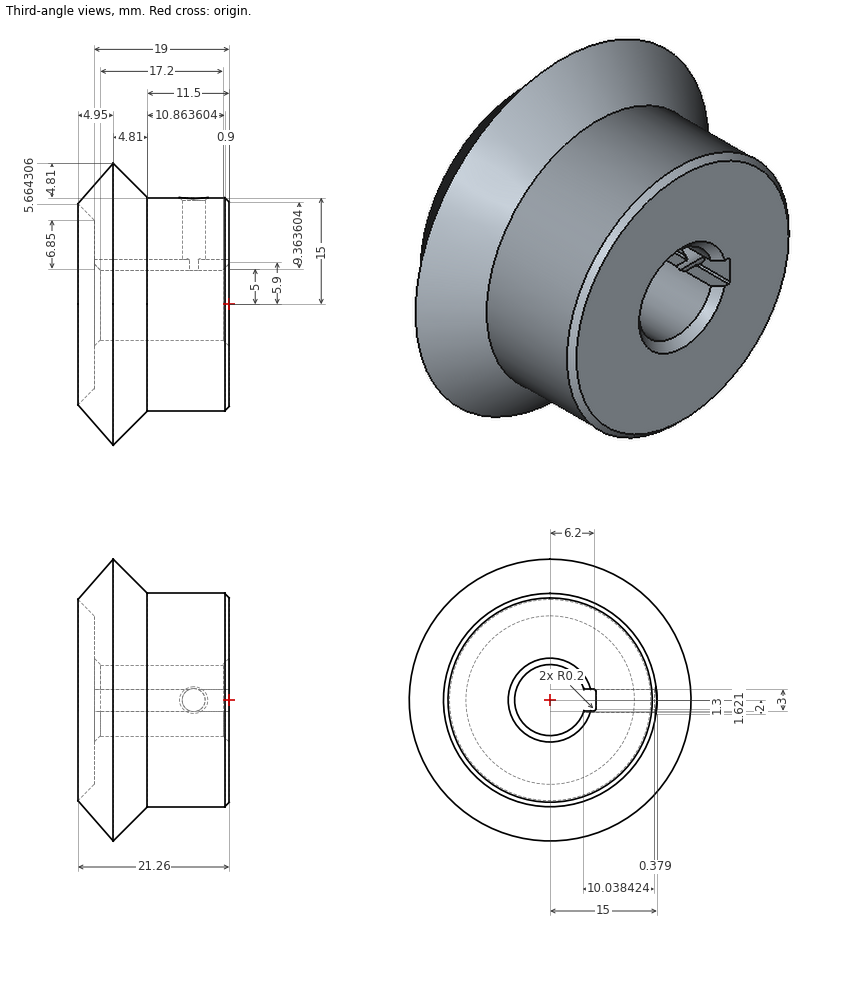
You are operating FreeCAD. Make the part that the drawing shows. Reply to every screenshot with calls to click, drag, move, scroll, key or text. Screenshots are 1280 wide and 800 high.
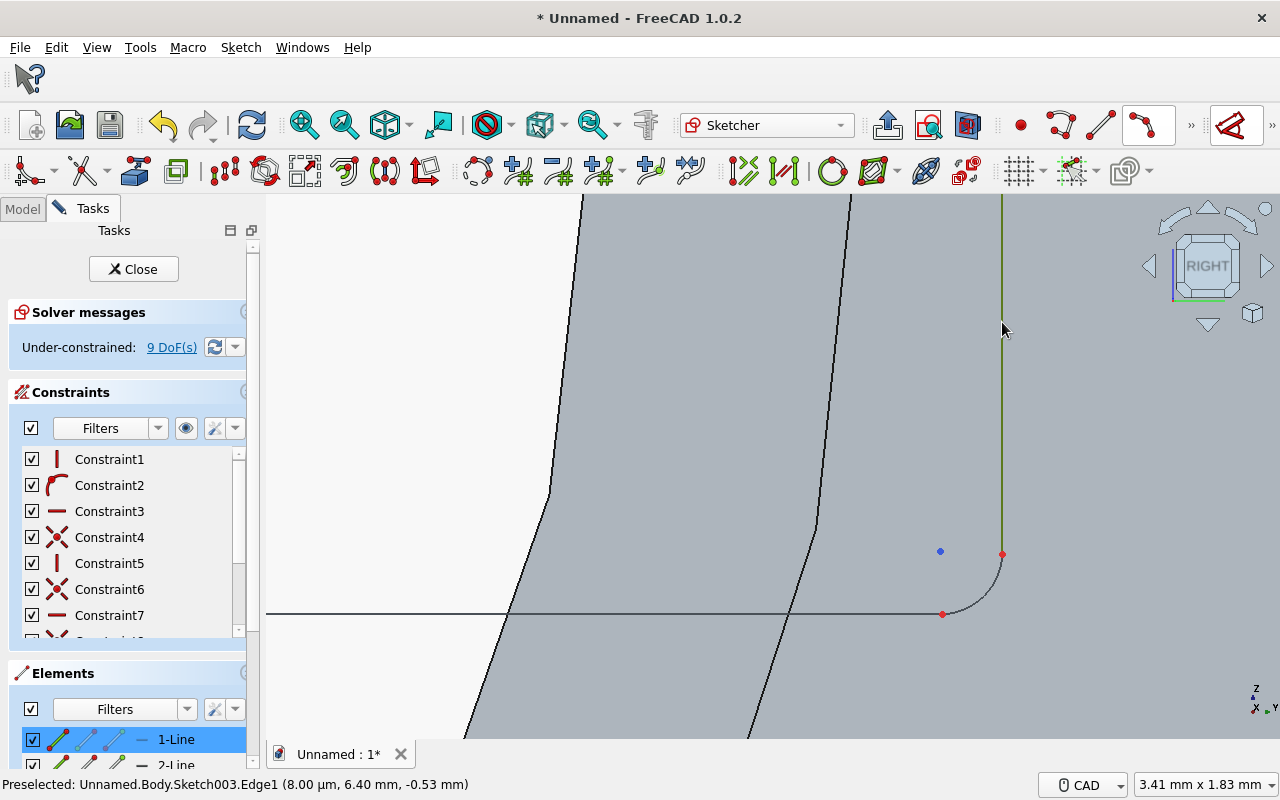
scroll(986, 597, down, 6)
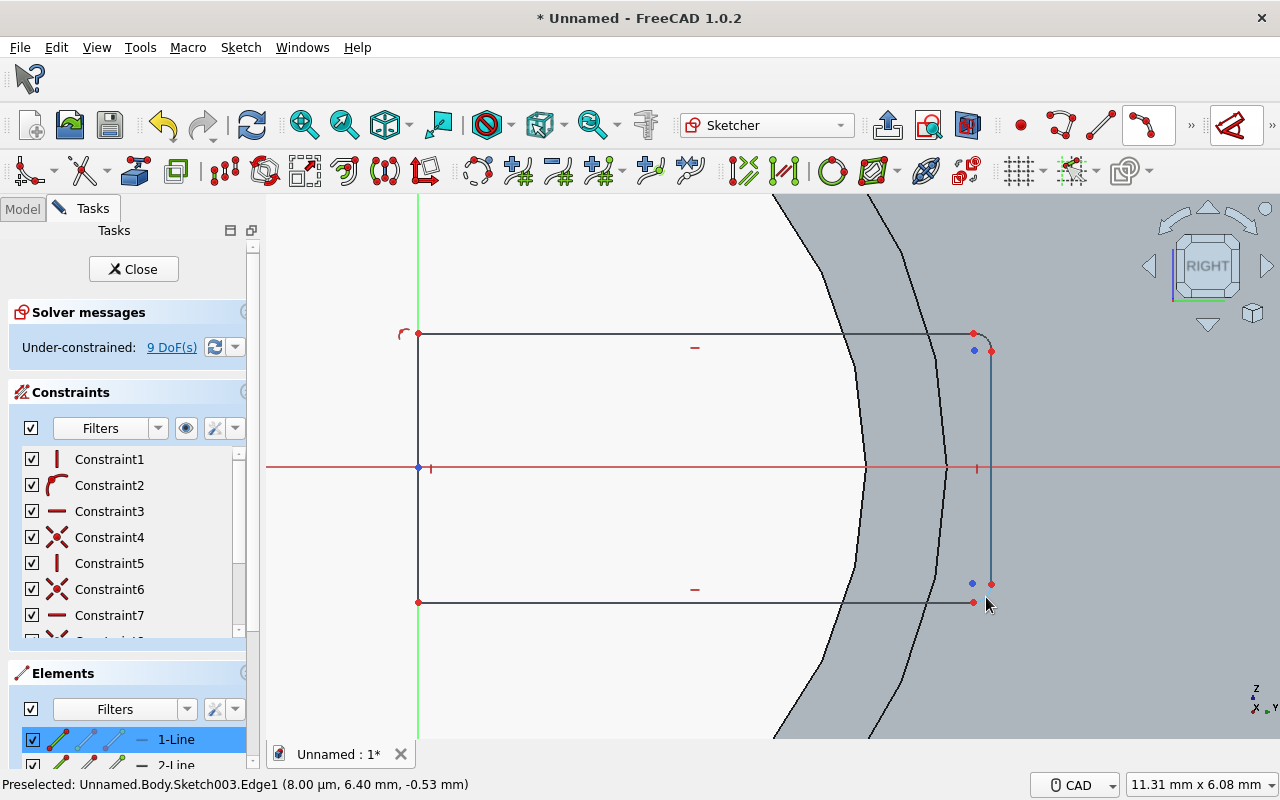
scroll(990, 343, up, 3)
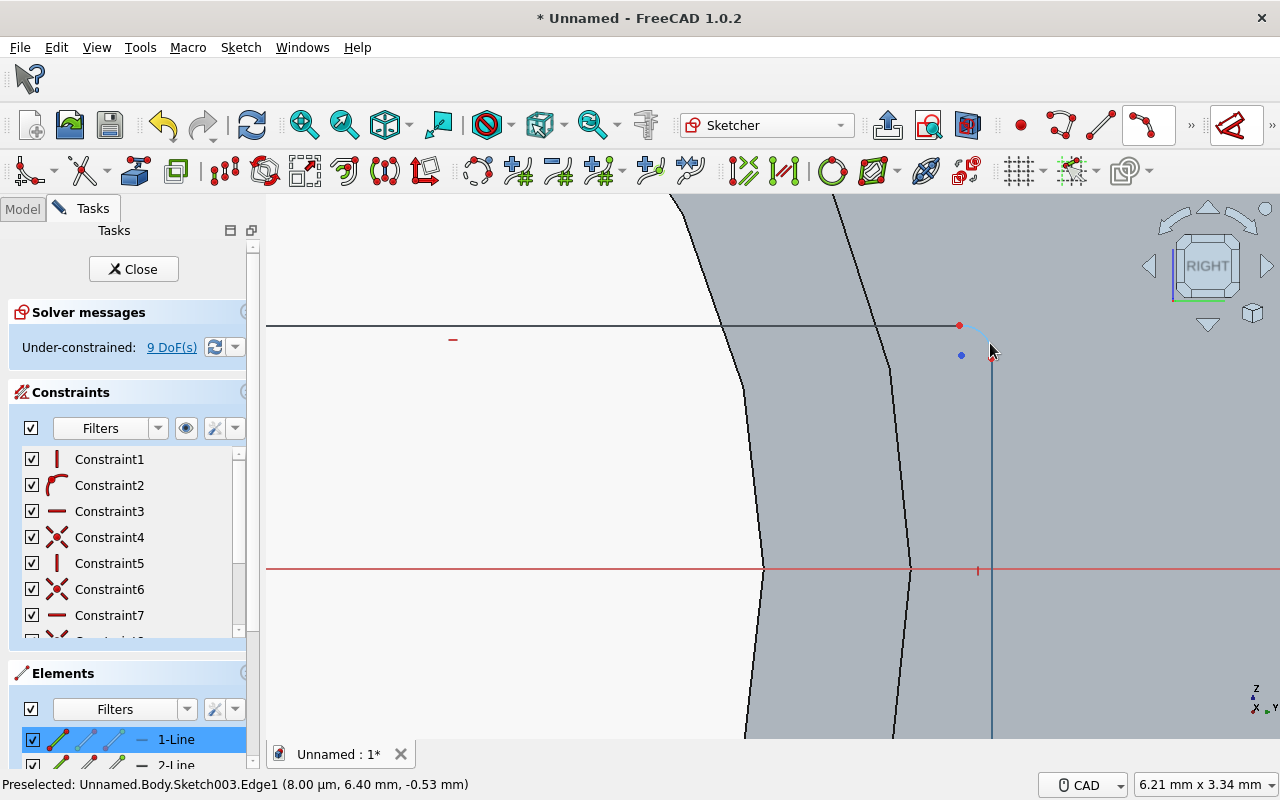
click(989, 343)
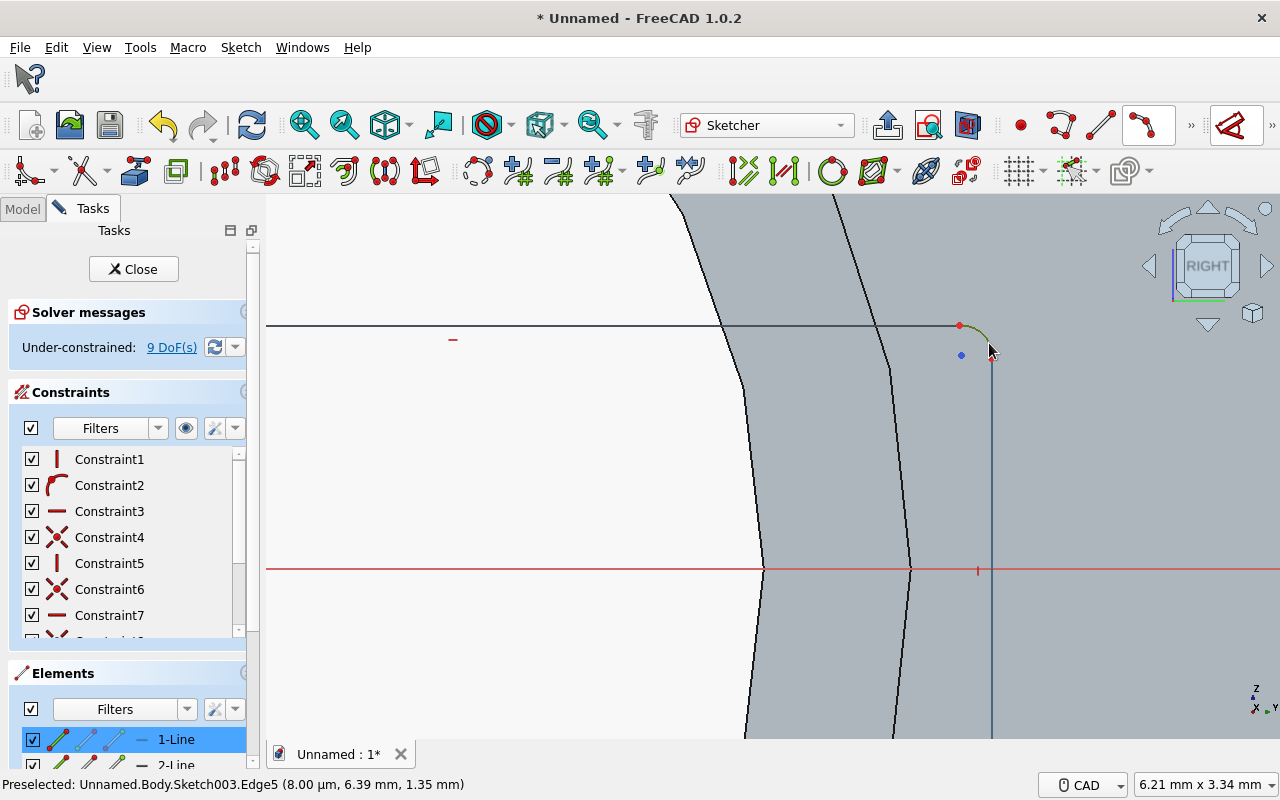
key(t)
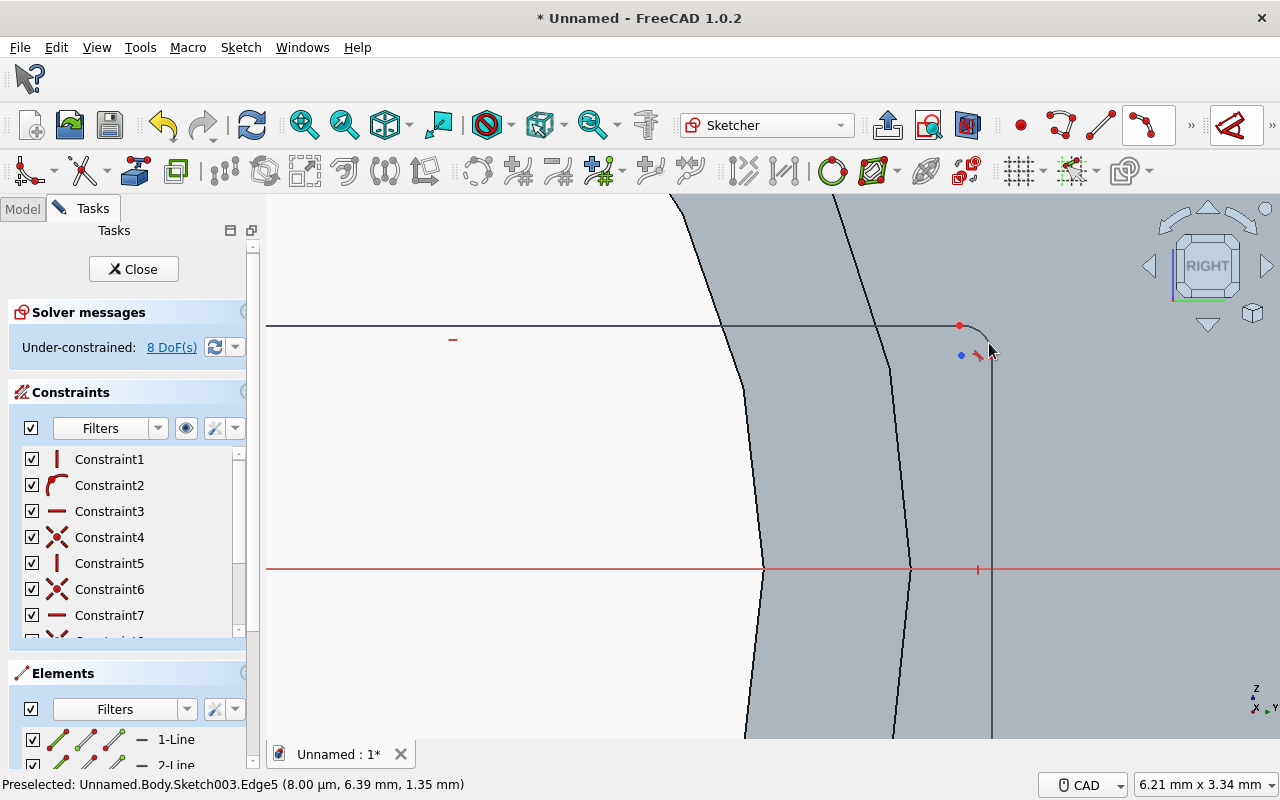
click(992, 655)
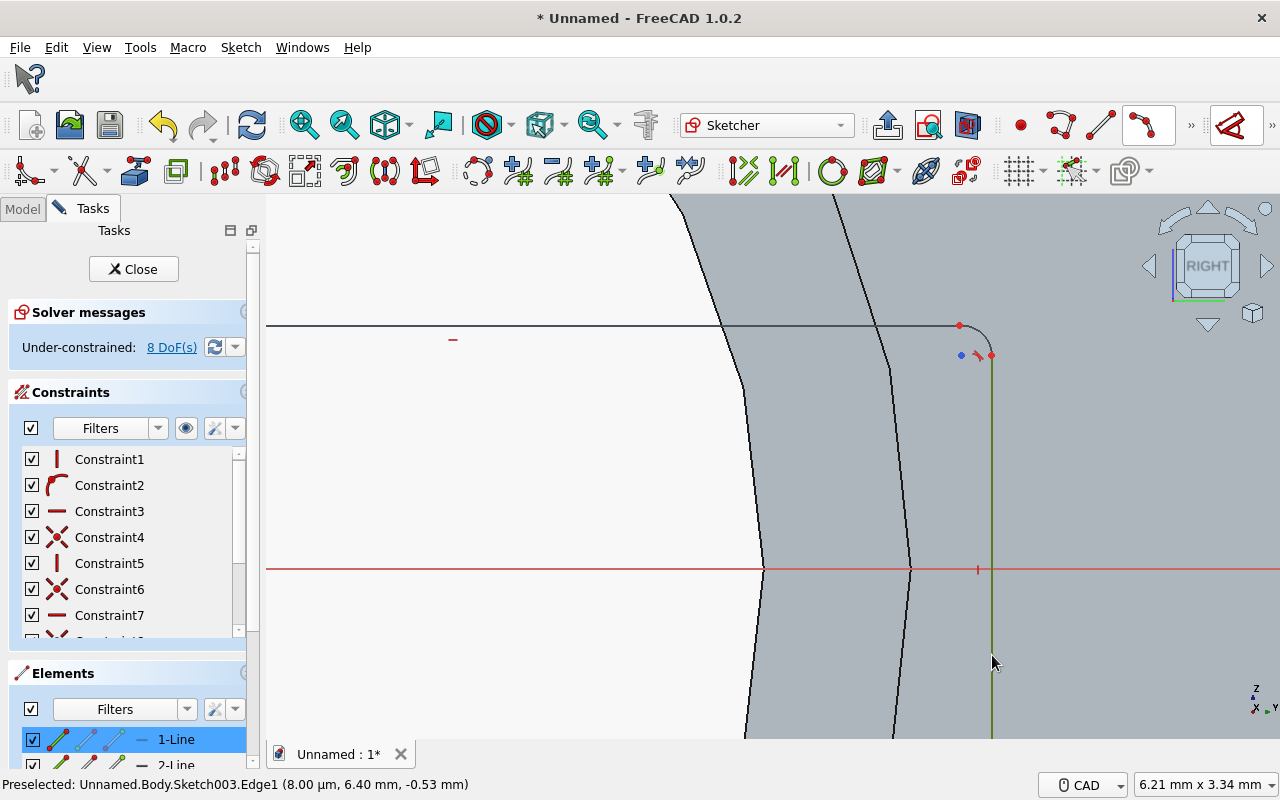
scroll(990, 342, down, 3)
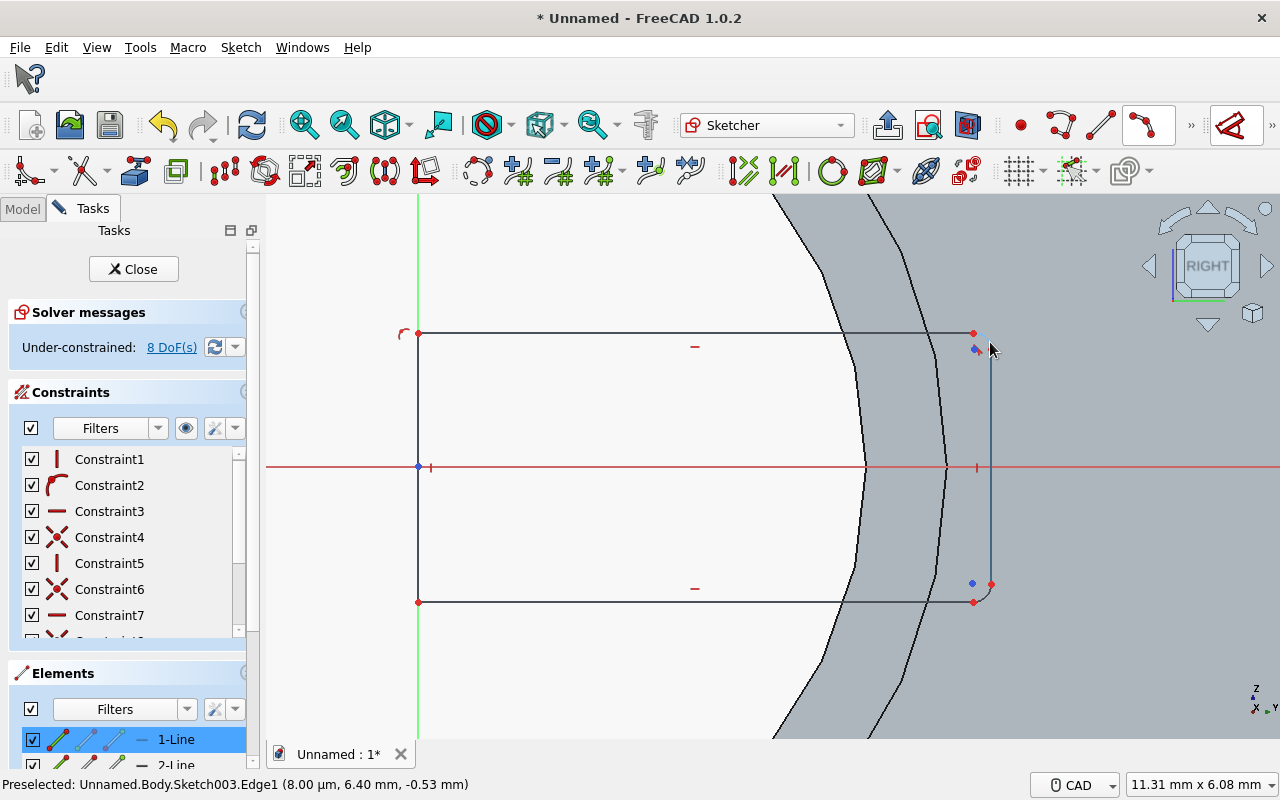
scroll(981, 600, up, 3)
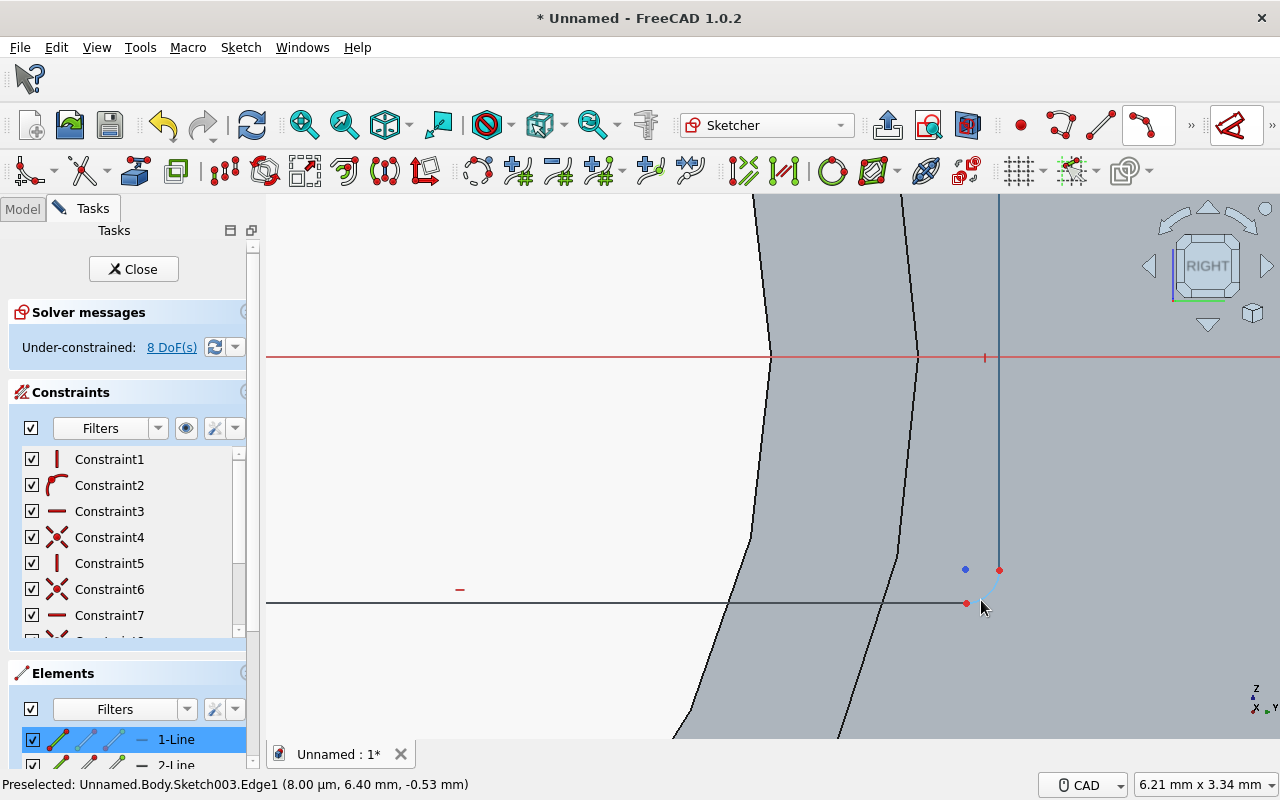
click(981, 600)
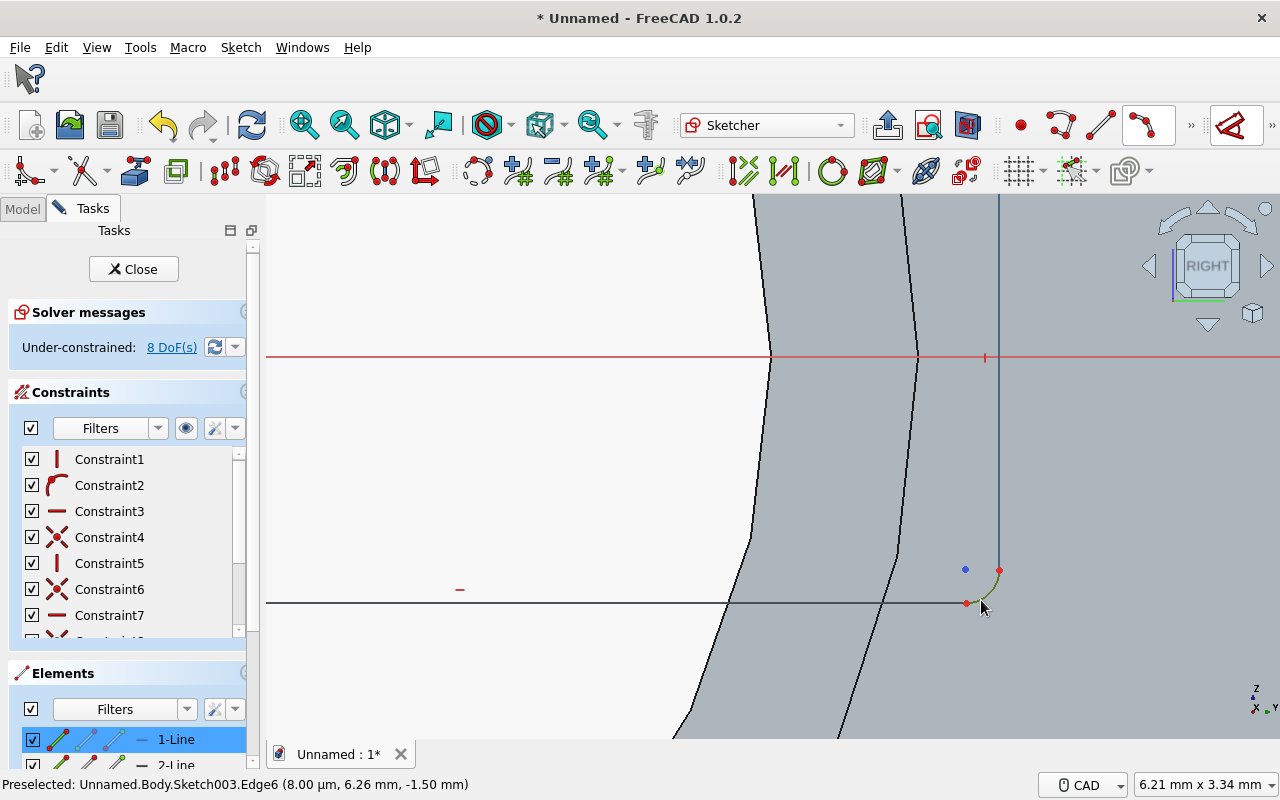
key(t)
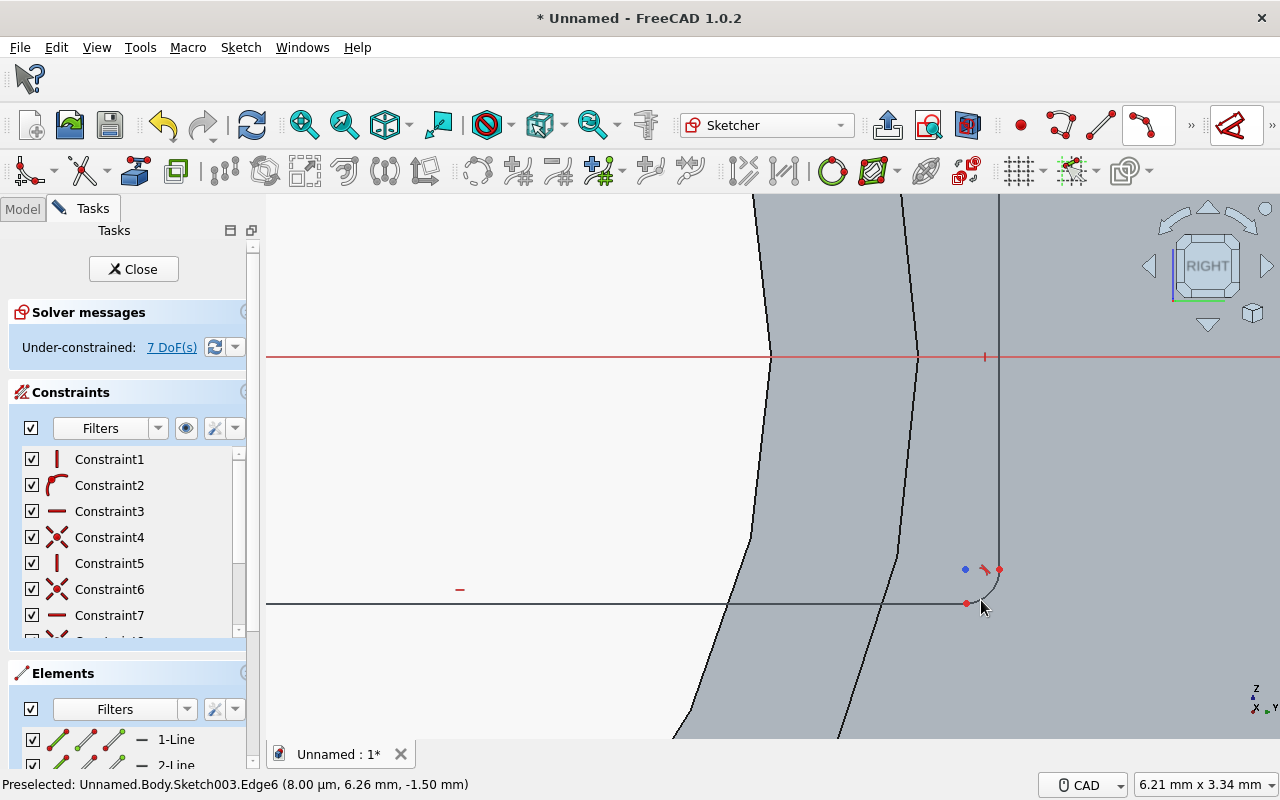
scroll(981, 600, down, 3)